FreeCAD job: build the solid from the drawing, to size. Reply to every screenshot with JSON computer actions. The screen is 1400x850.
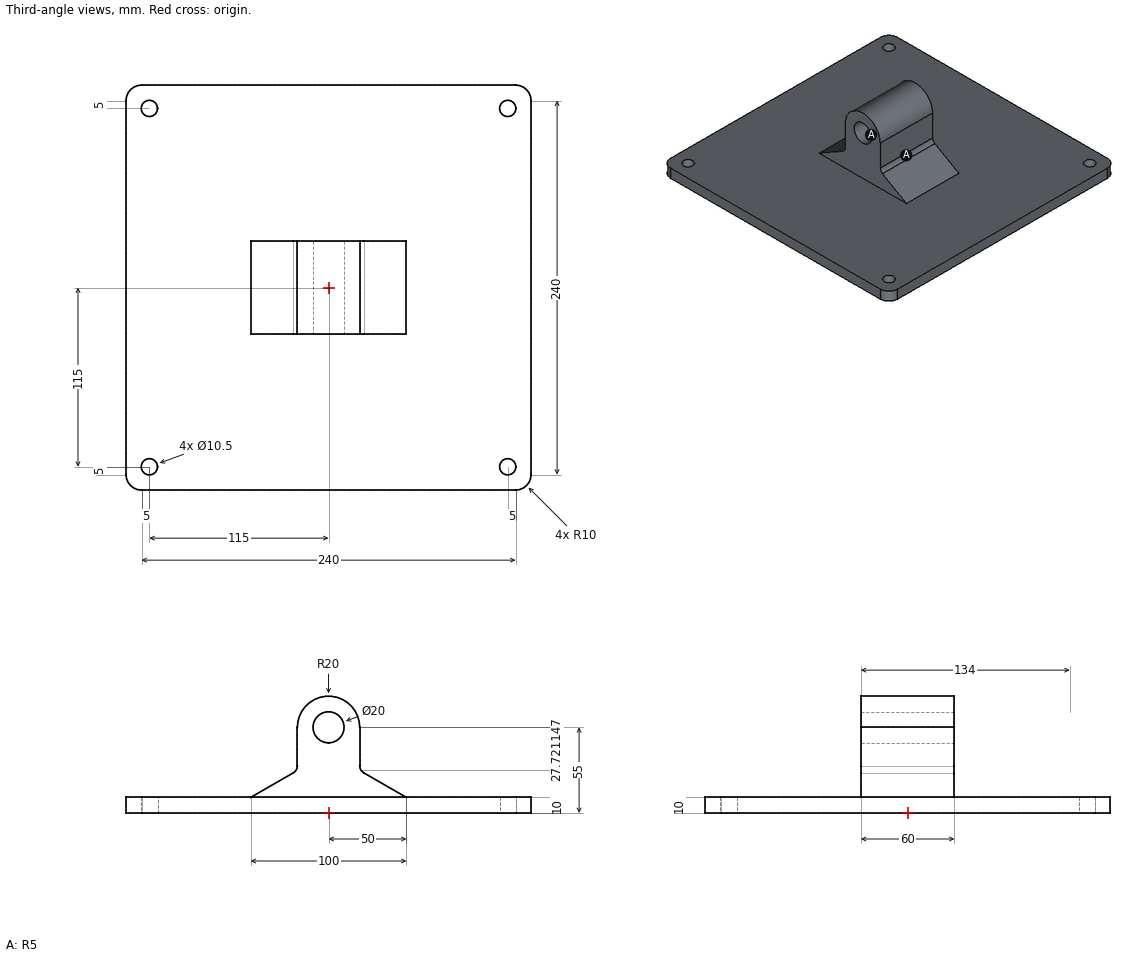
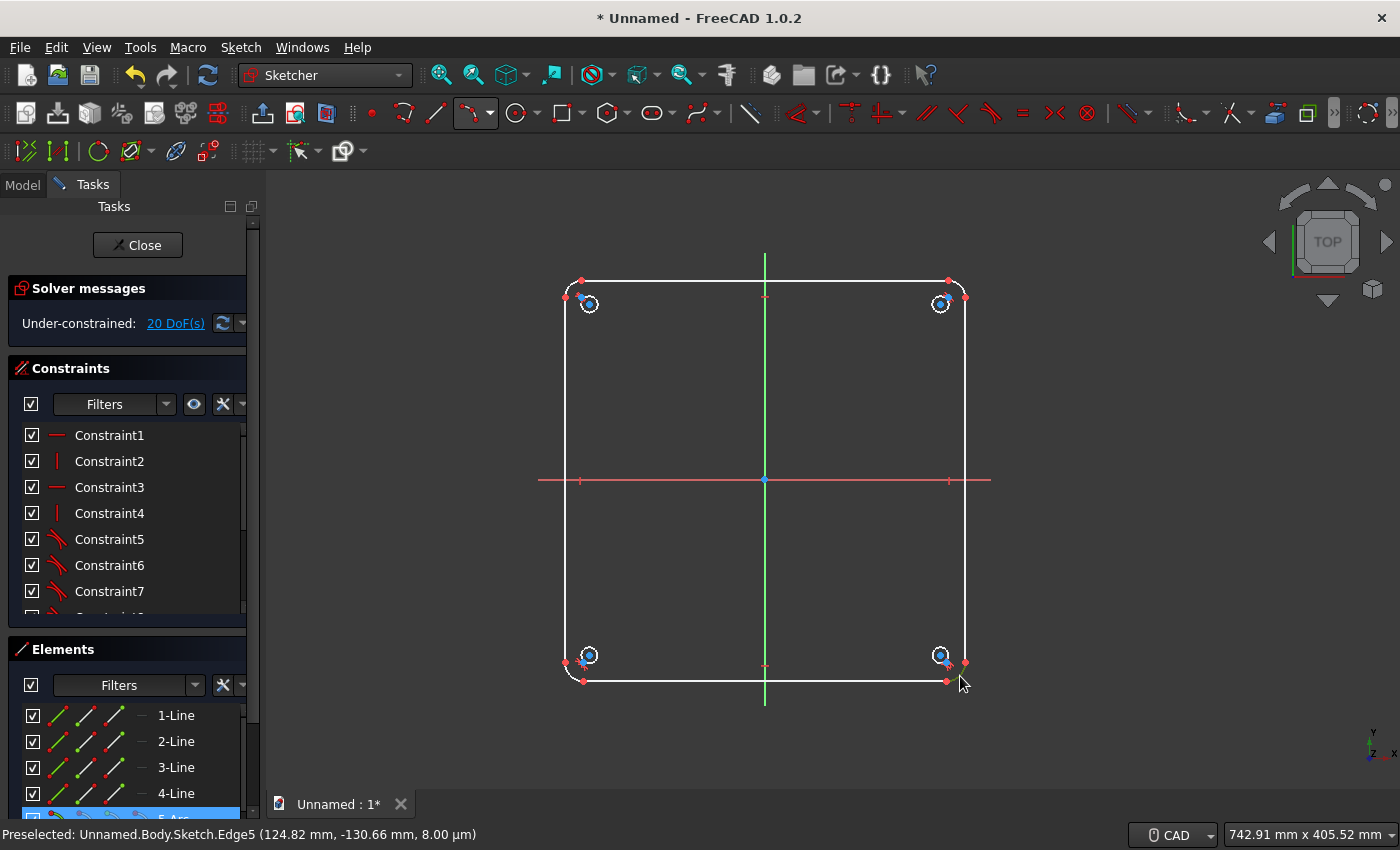
{"action": "left_click", "coordinate": [960, 286]}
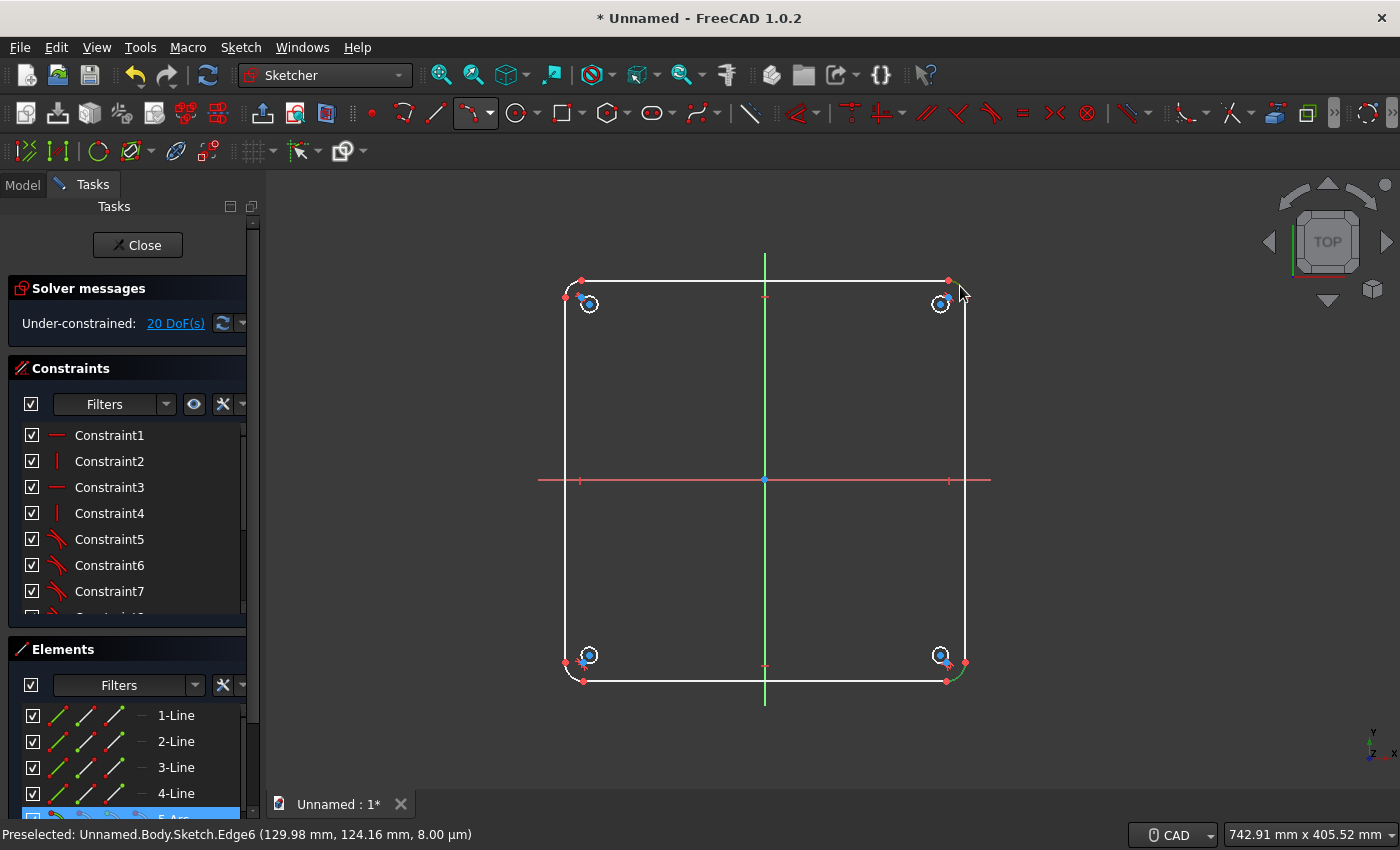
{"action": "left_click", "coordinate": [570, 286]}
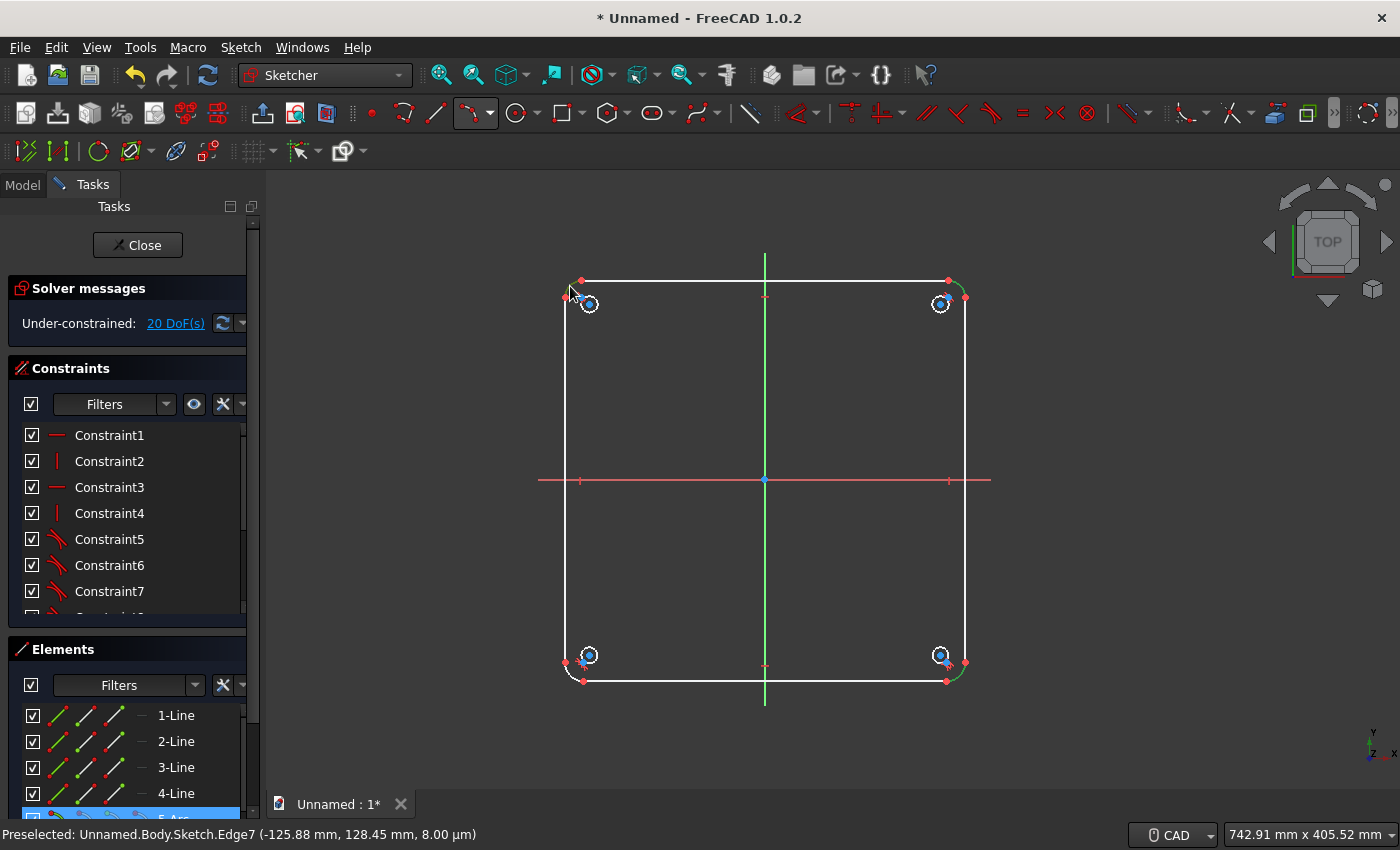
{"action": "left_click", "coordinate": [571, 676]}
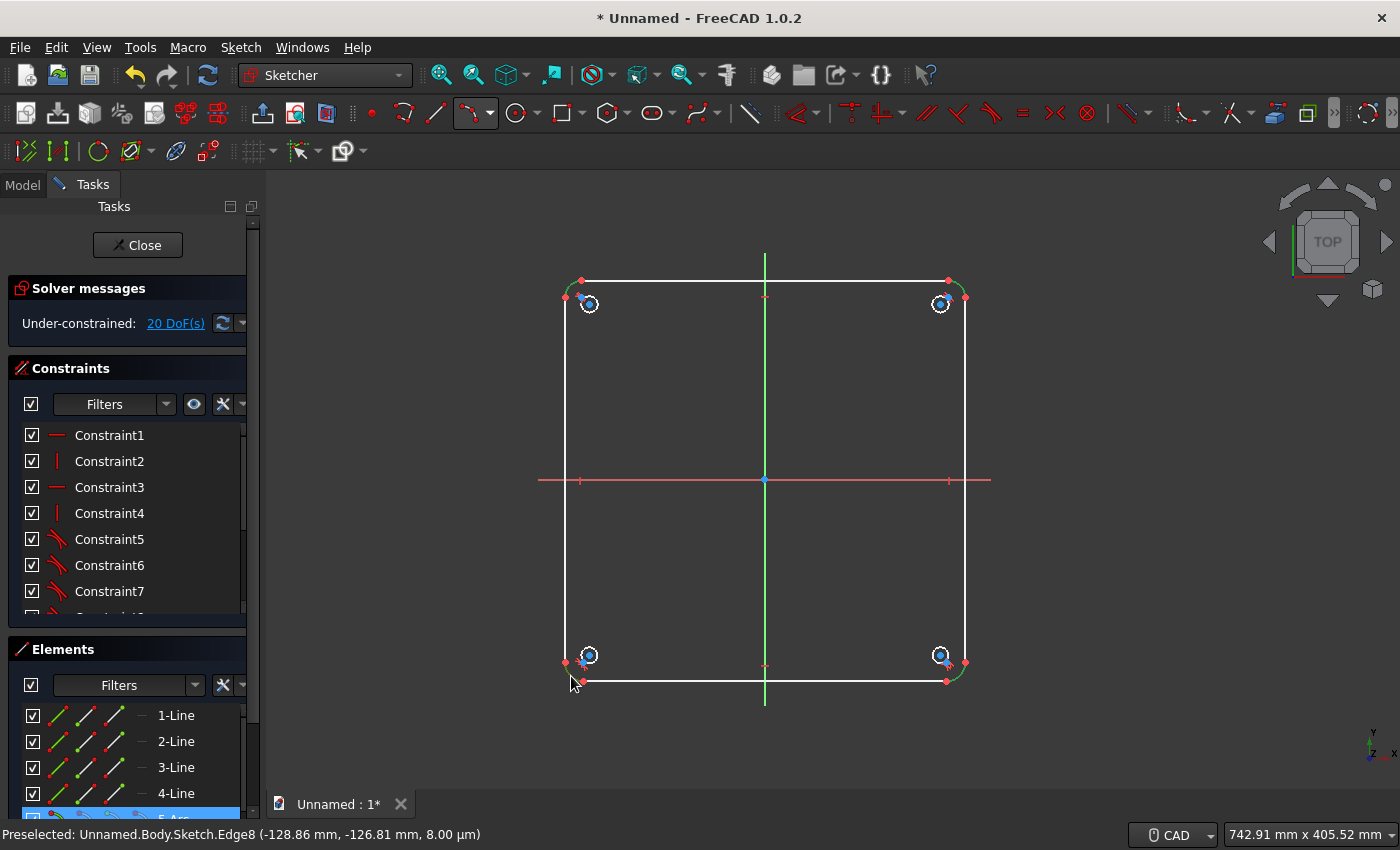
{"action": "left_click", "coordinate": [1024, 114]}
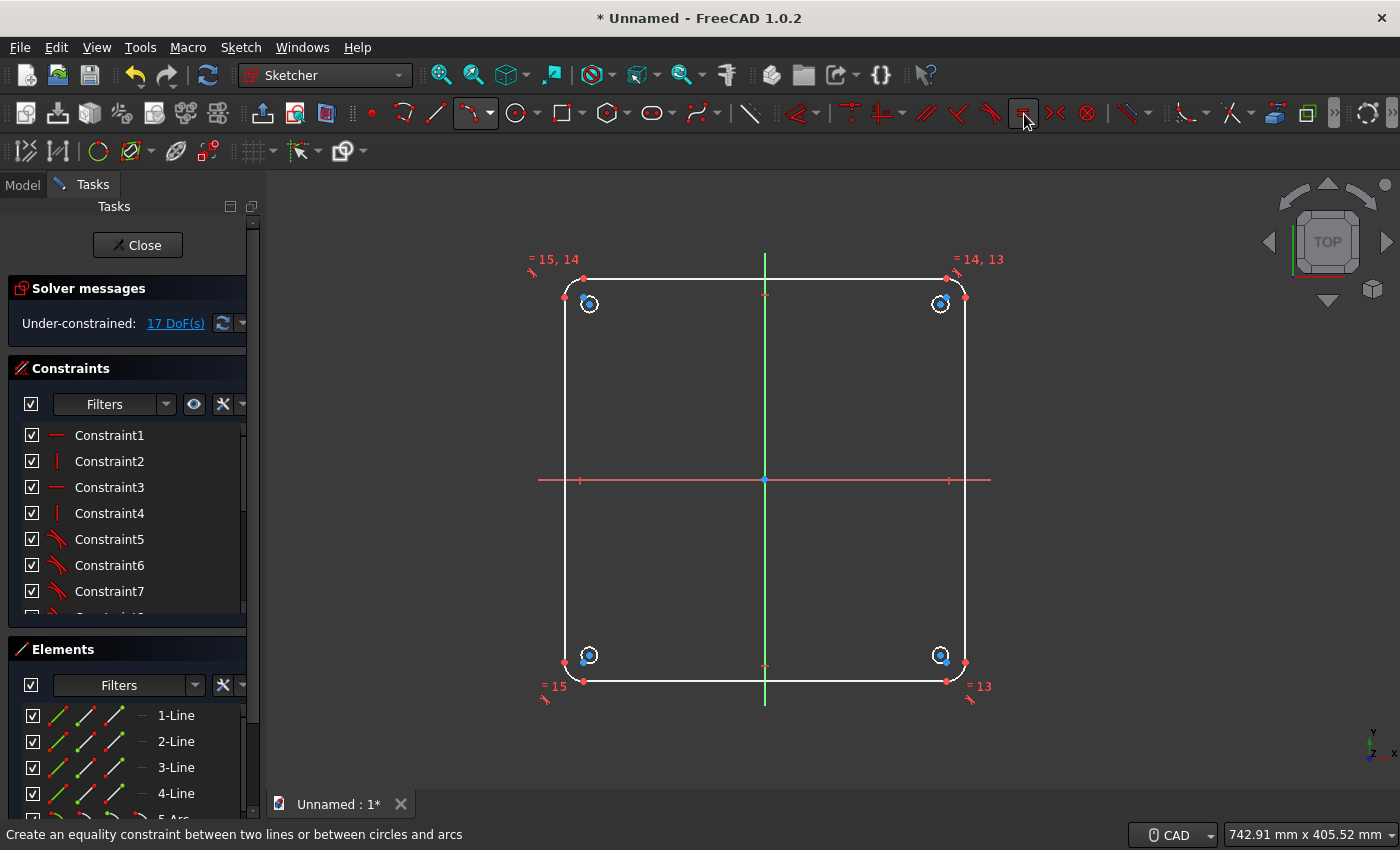
{"action": "scroll", "coordinate": [595, 661], "scroll_direction": "up", "scroll_amount": 3}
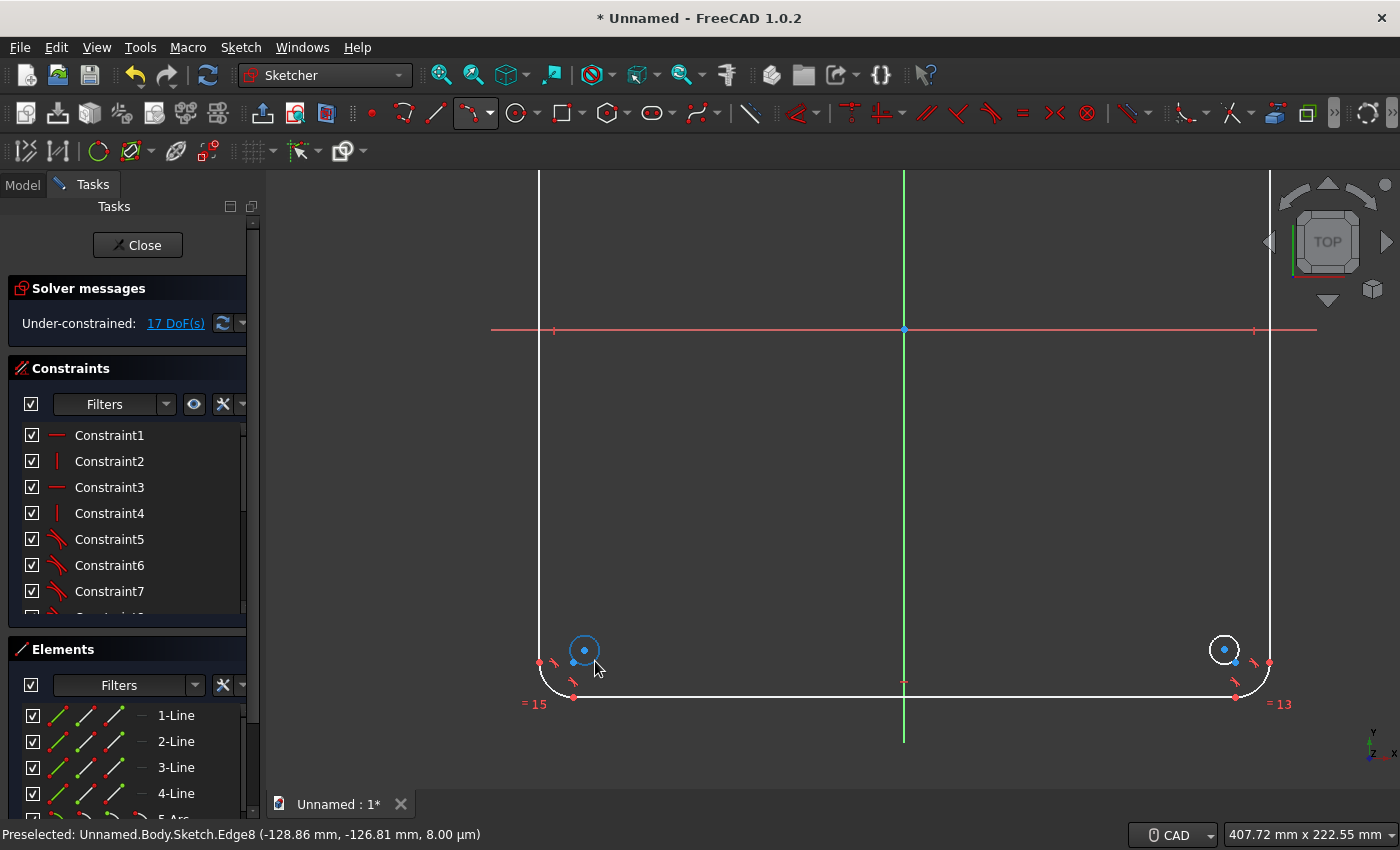
{"action": "left_click", "coordinate": [595, 660]}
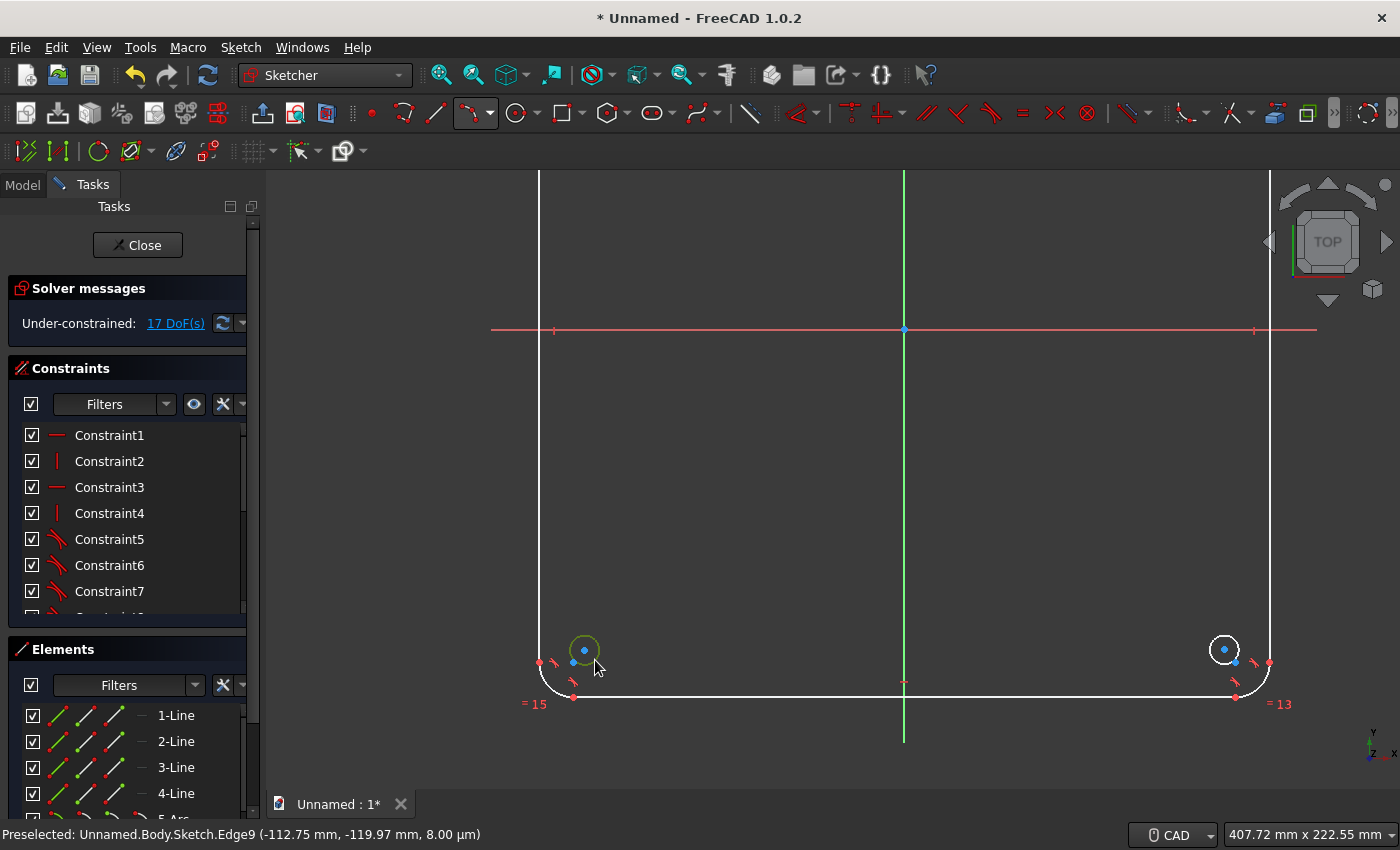
{"action": "left_click", "coordinate": [1234, 640]}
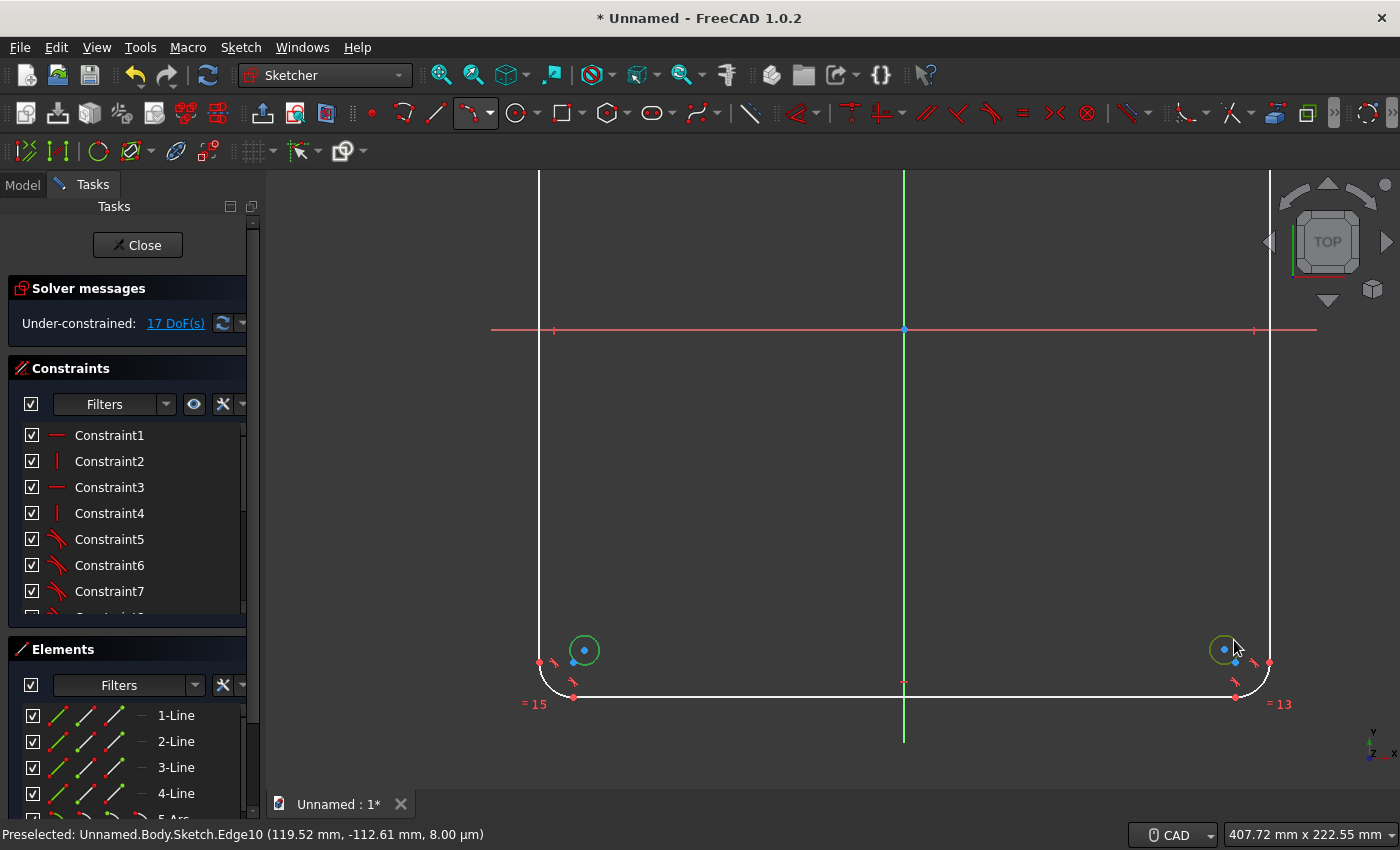
{"action": "scroll", "coordinate": [594, 662], "scroll_direction": "down", "scroll_amount": 3}